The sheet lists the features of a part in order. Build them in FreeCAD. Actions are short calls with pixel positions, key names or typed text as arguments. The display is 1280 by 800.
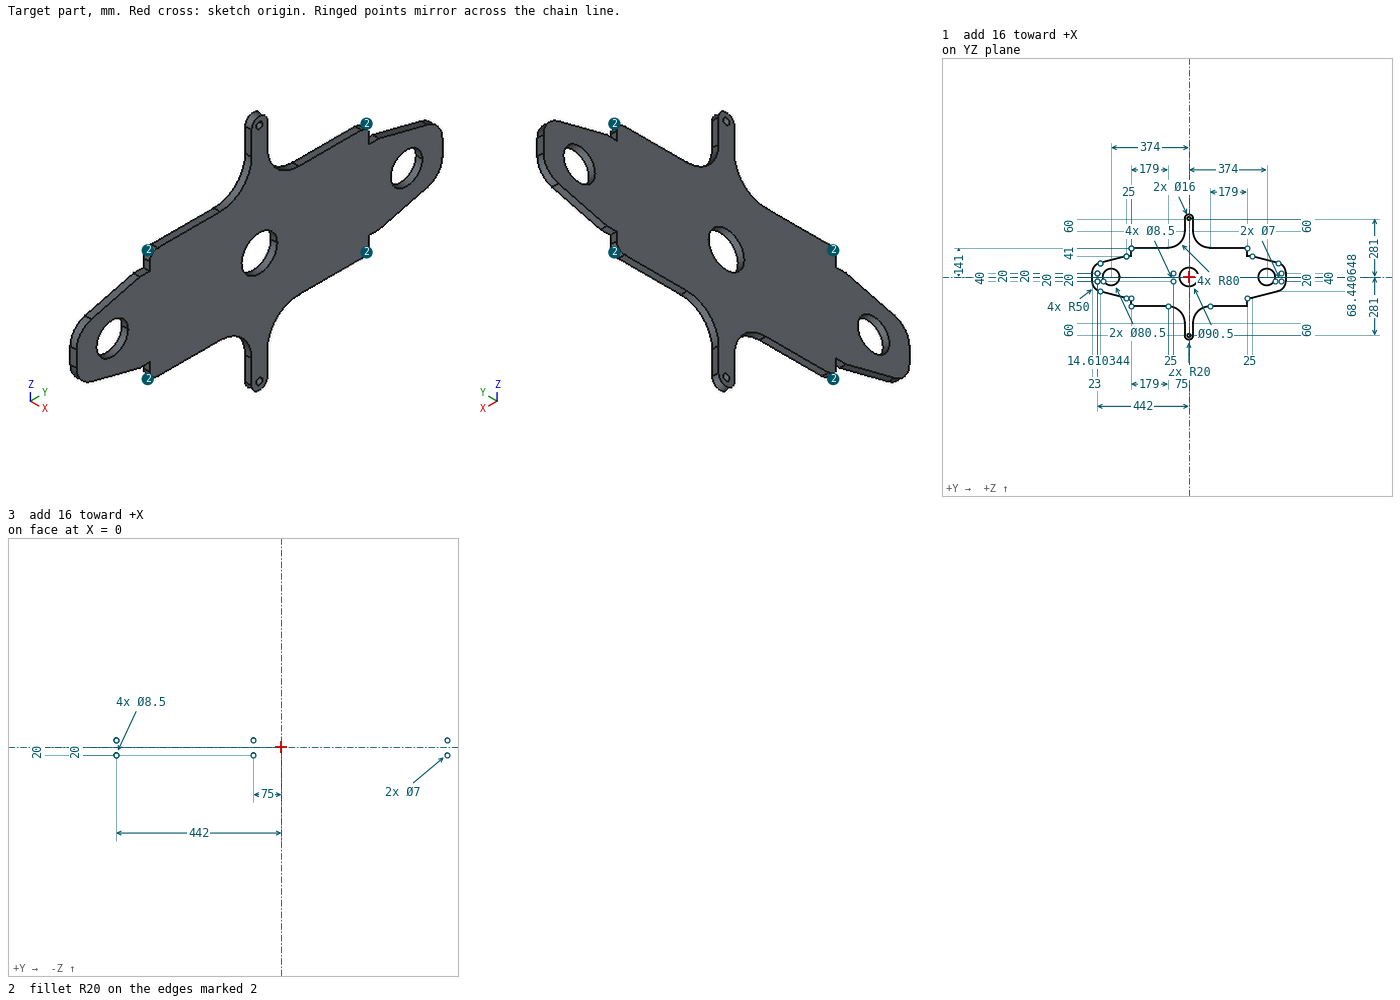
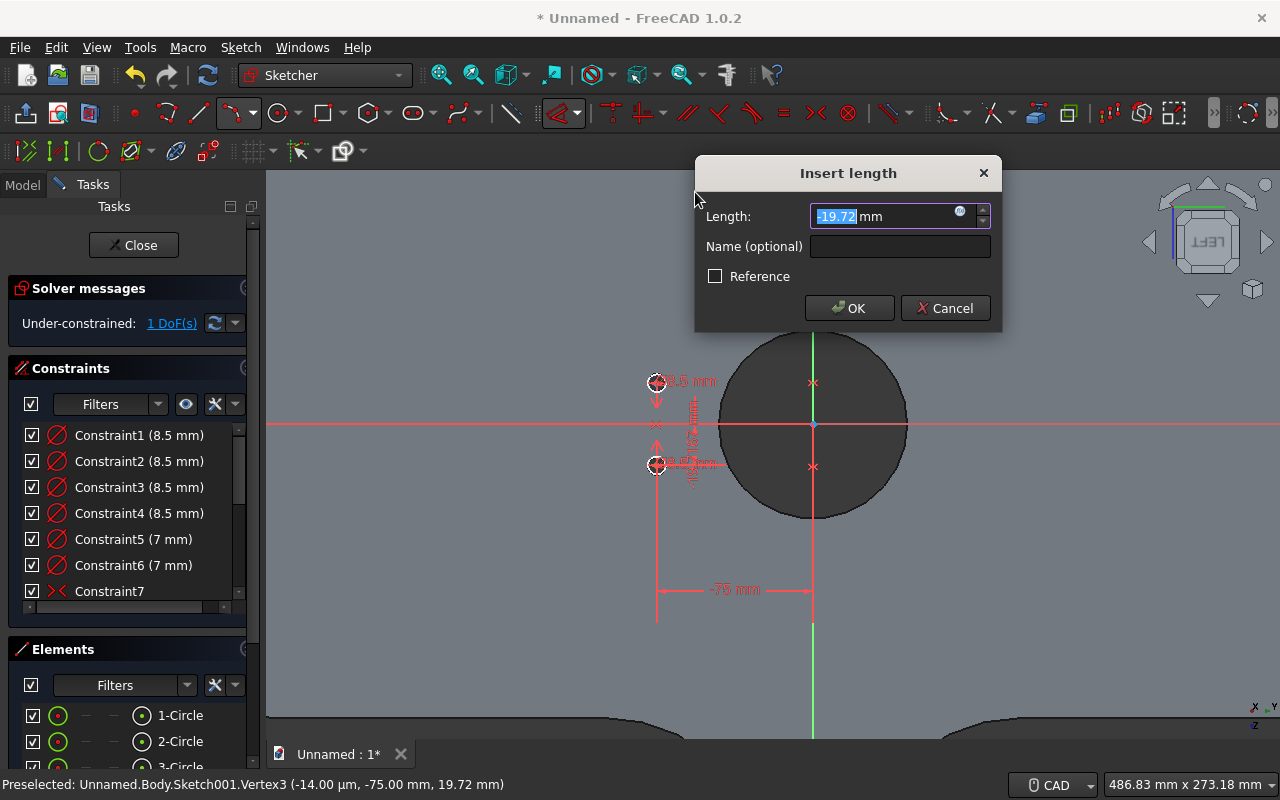
text(-20)
key(Return)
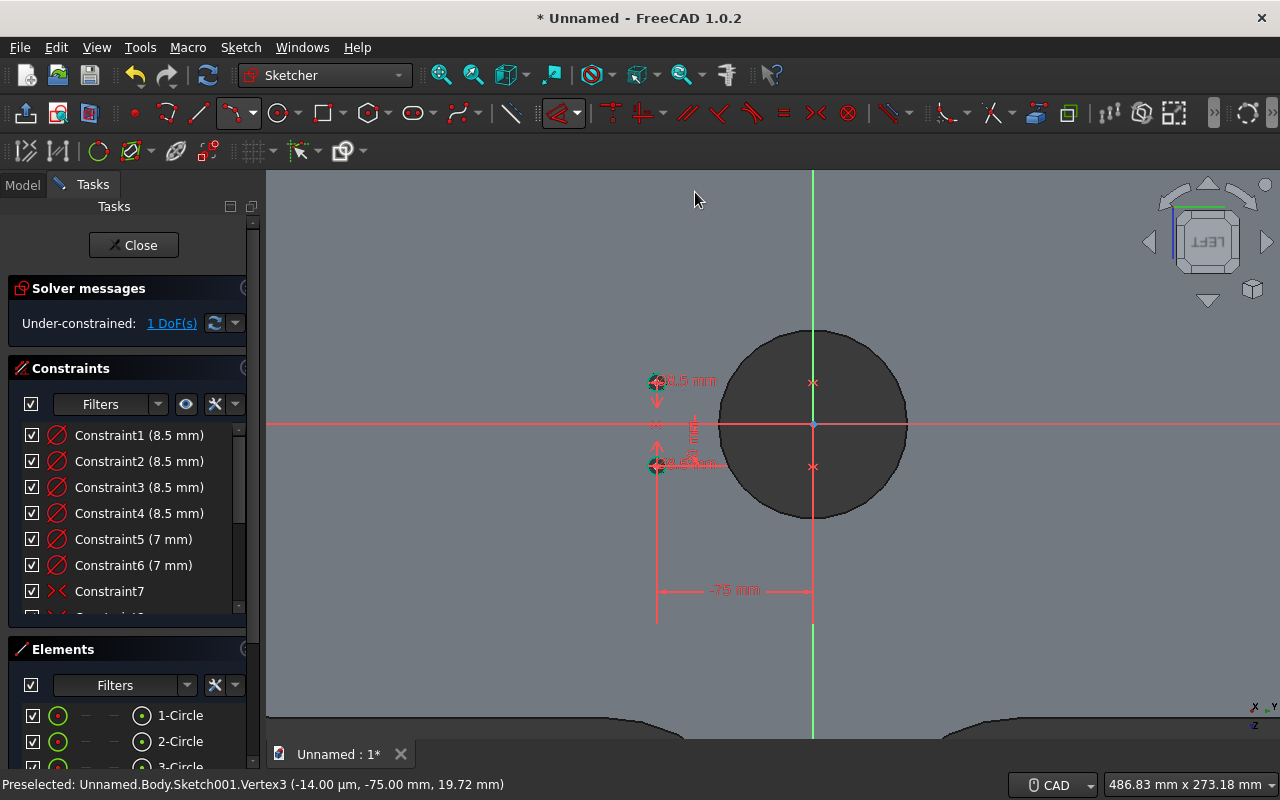
scroll(658, 467, down, 6)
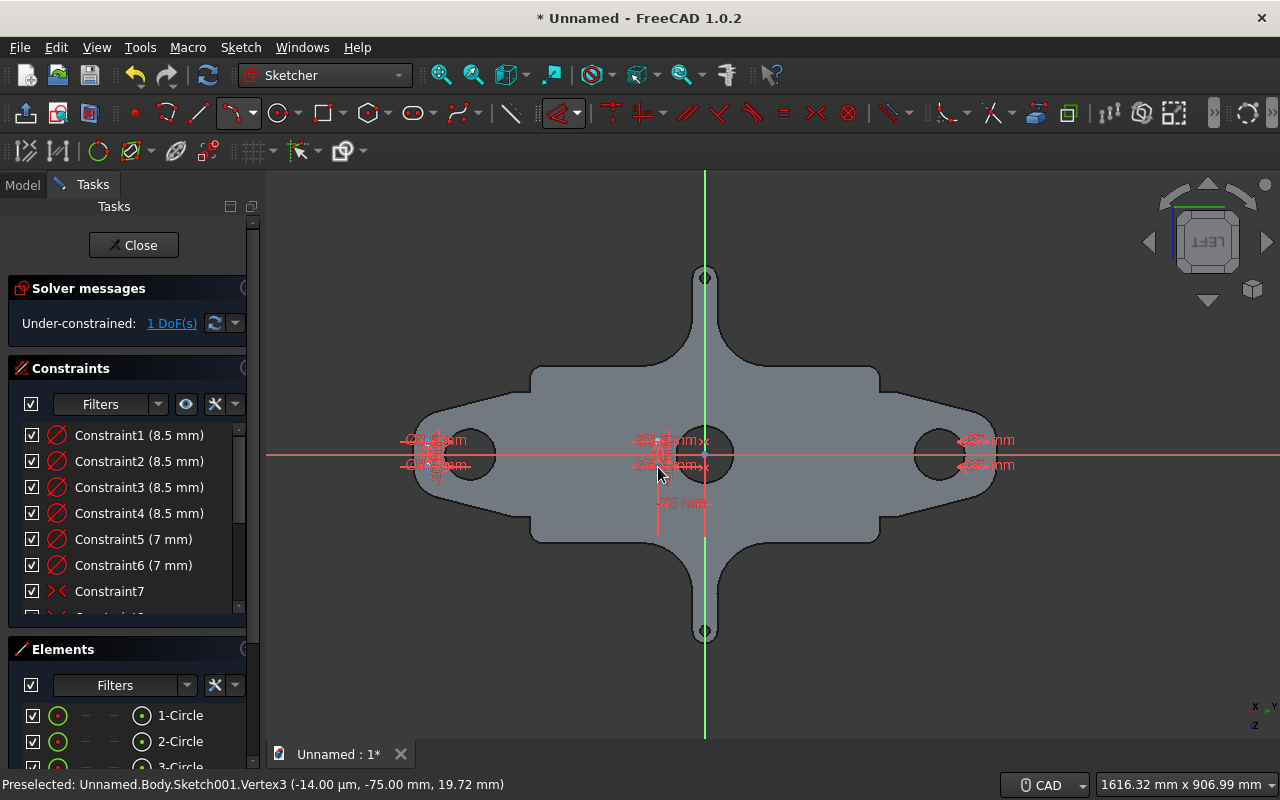
click(428, 467)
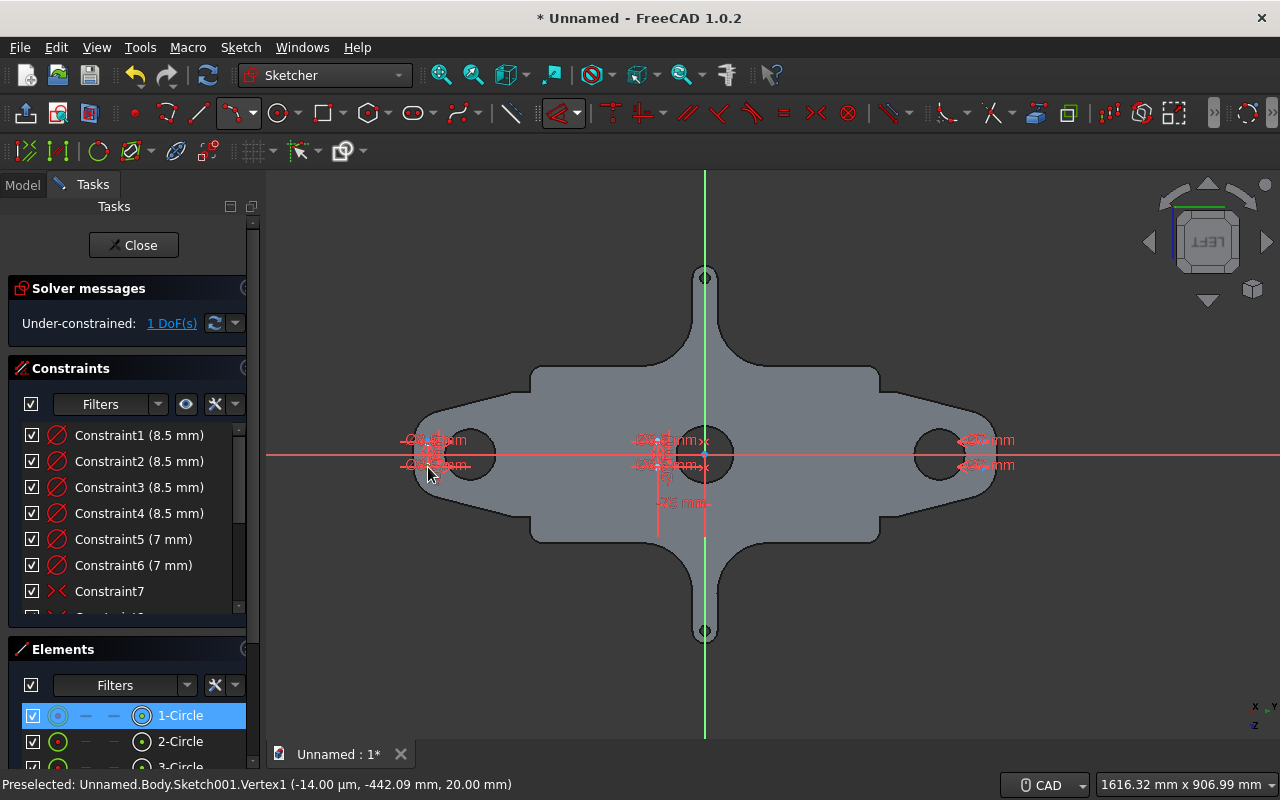
key(l)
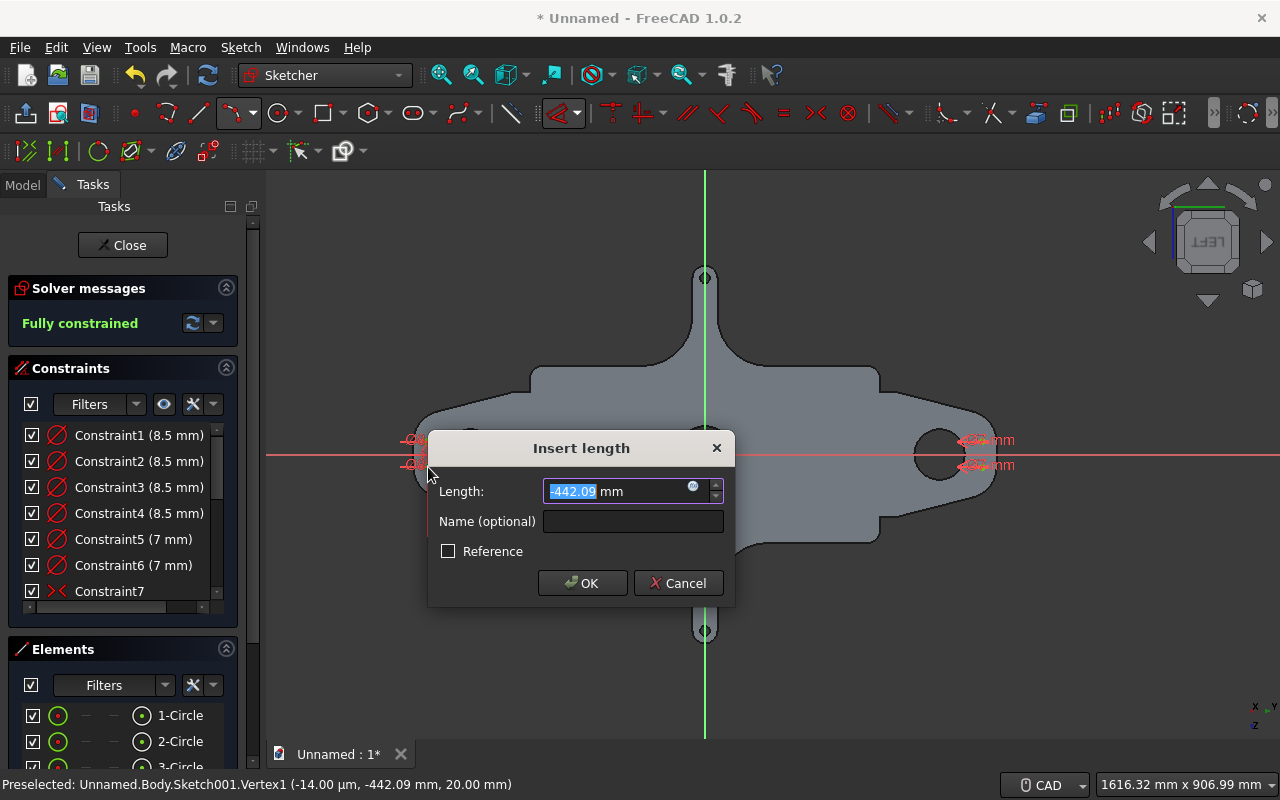
text(-442)
key(Return)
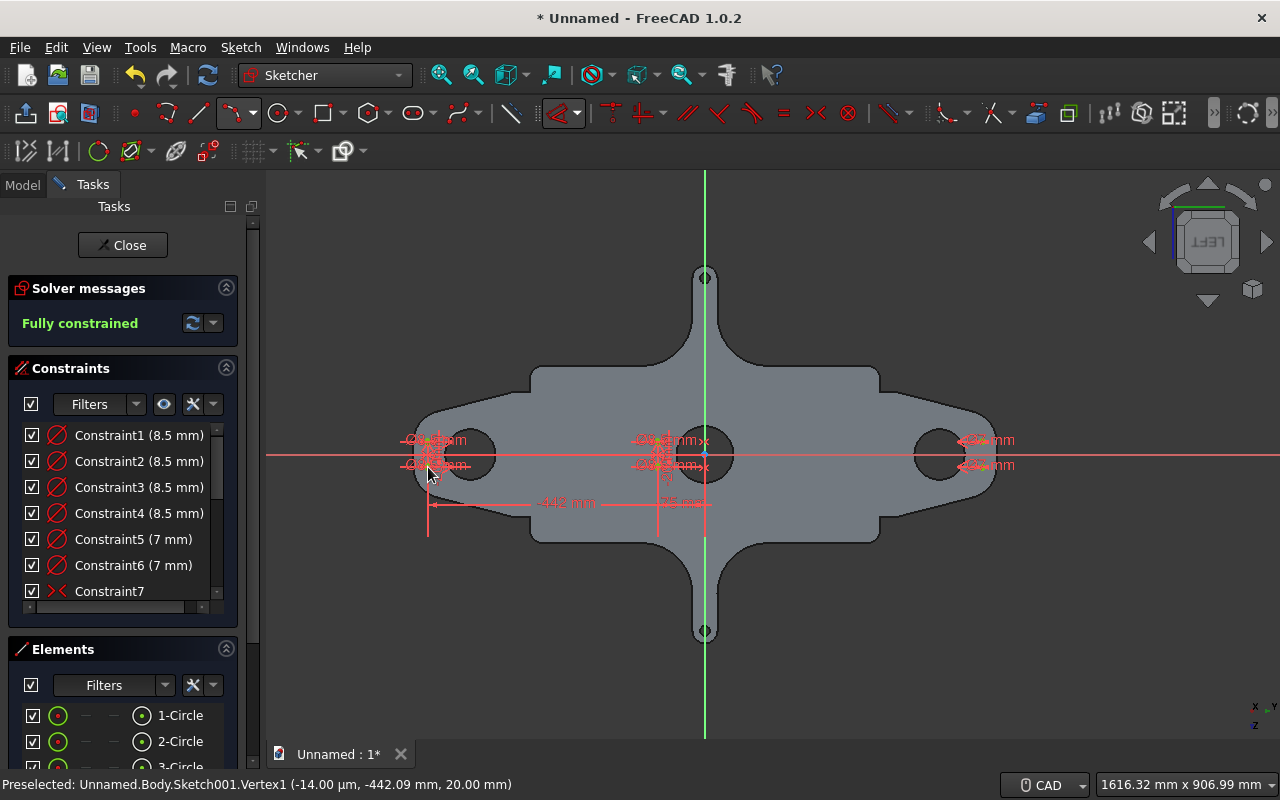
click(123, 245)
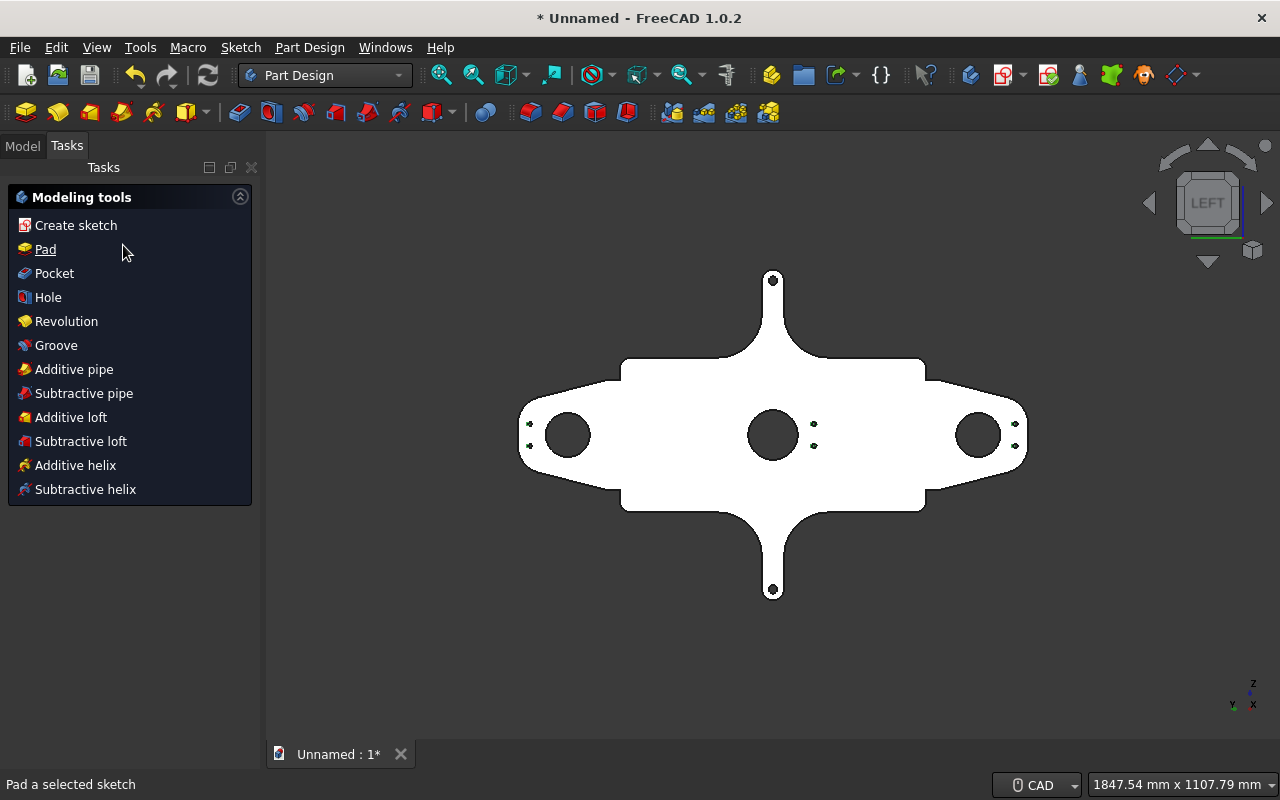
click(26, 112)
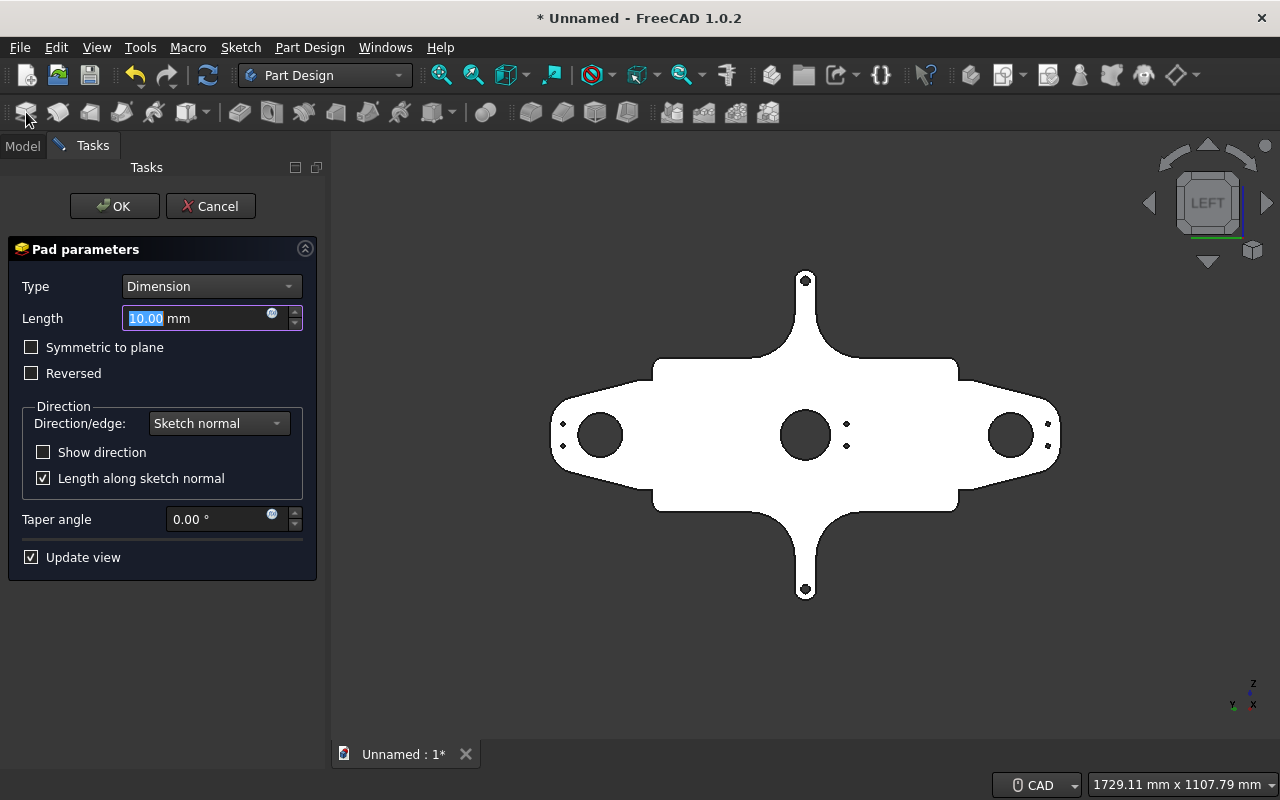
text(16)
key(Tab)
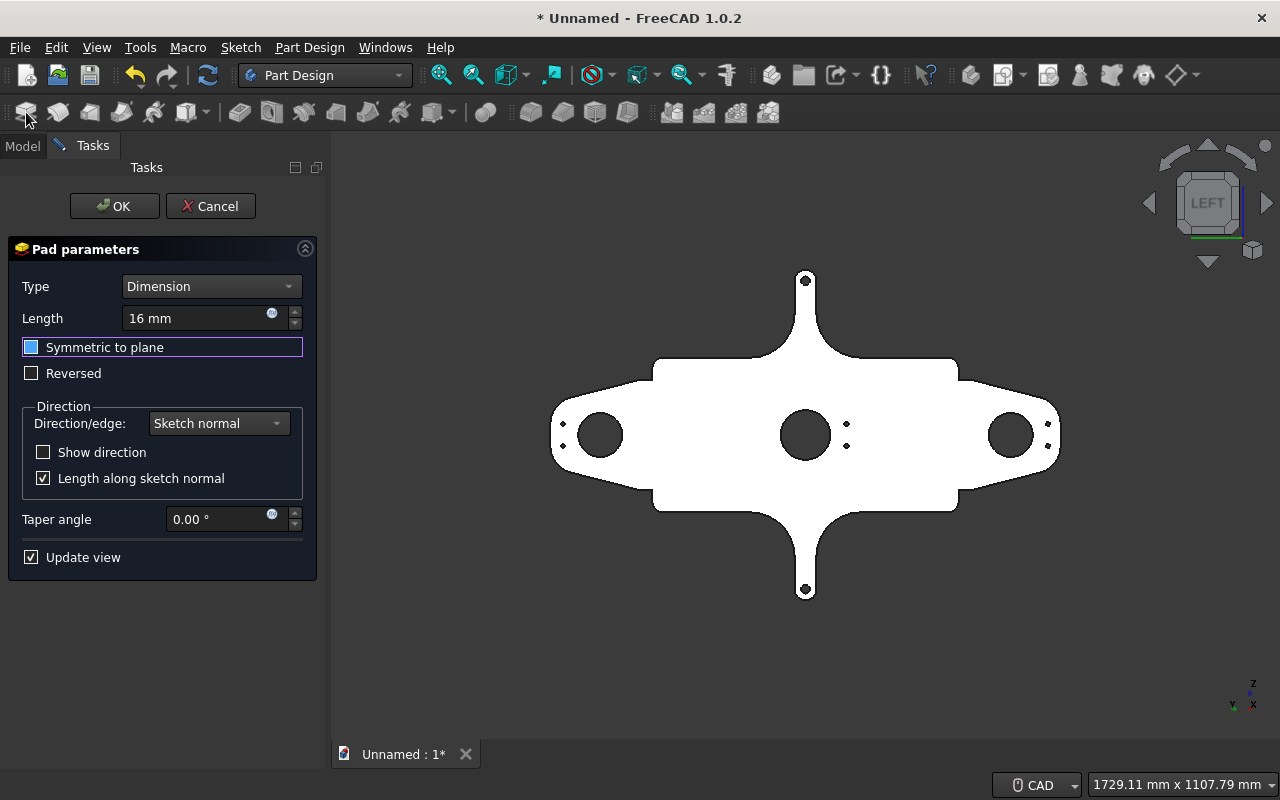
click(30, 373)